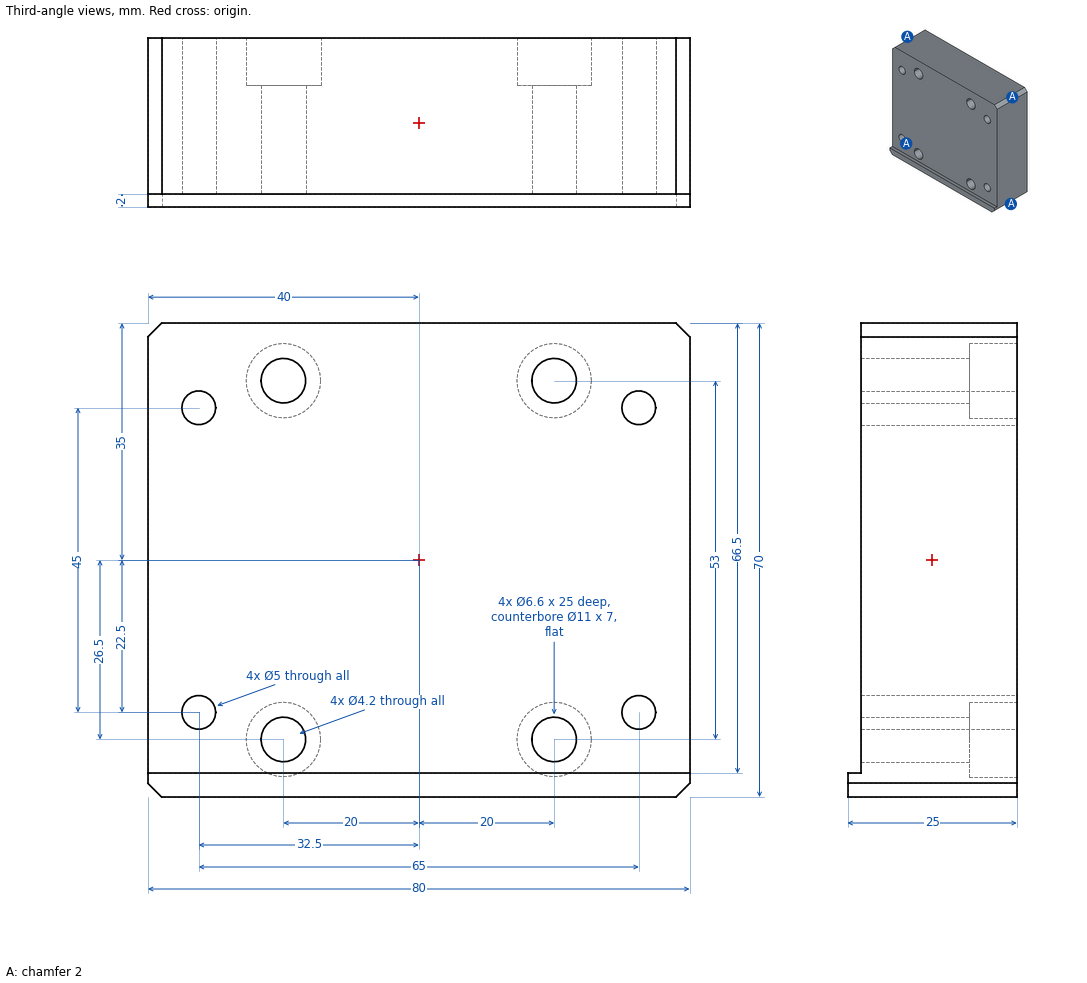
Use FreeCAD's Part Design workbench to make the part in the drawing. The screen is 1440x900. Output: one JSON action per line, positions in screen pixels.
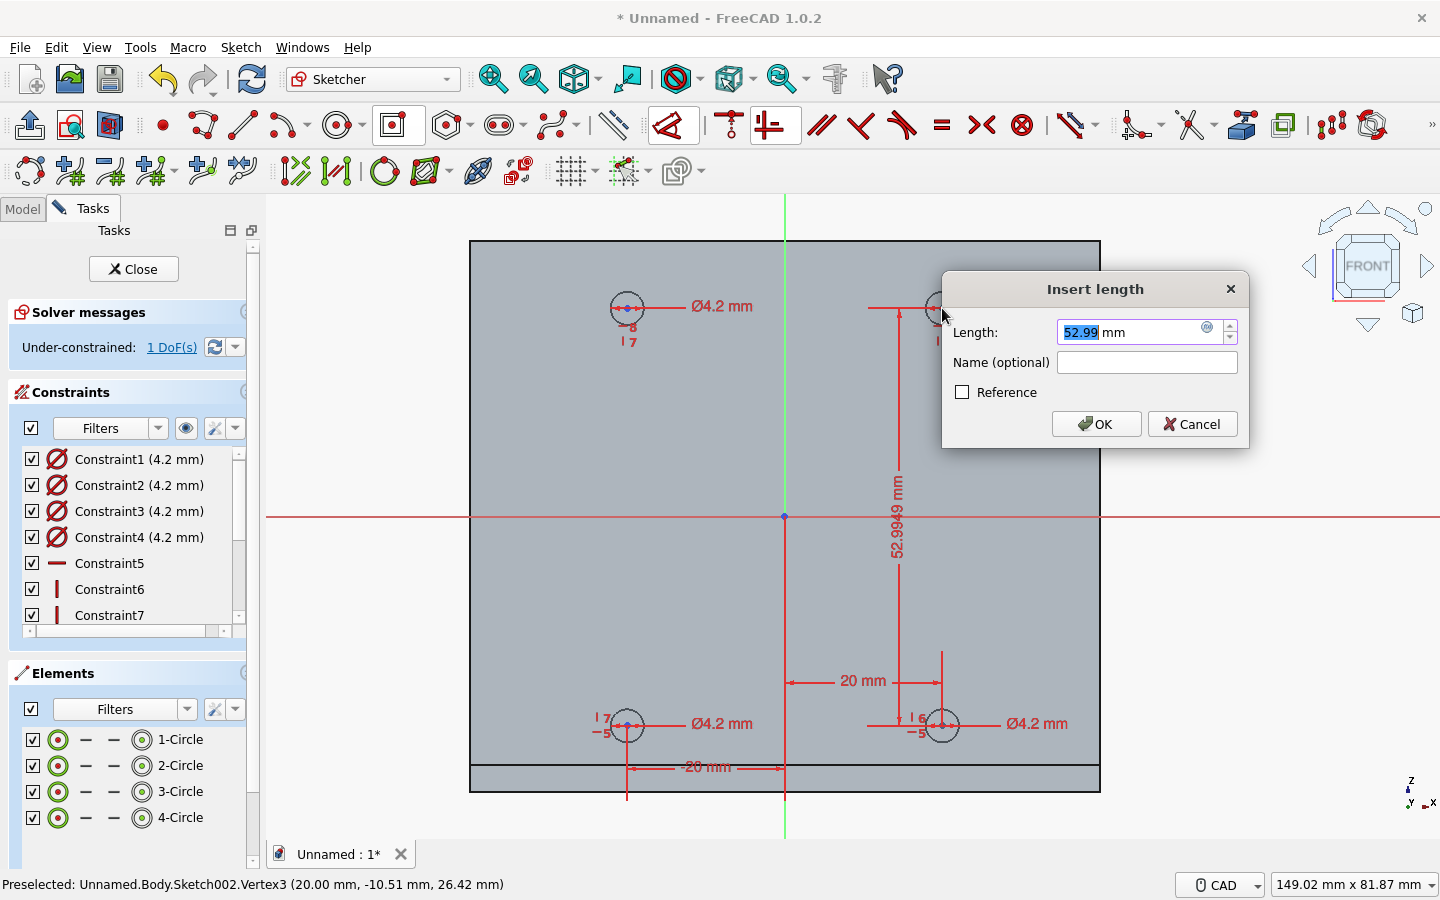
{"action": "type", "text": "53"}
{"action": "key", "text": "Return"}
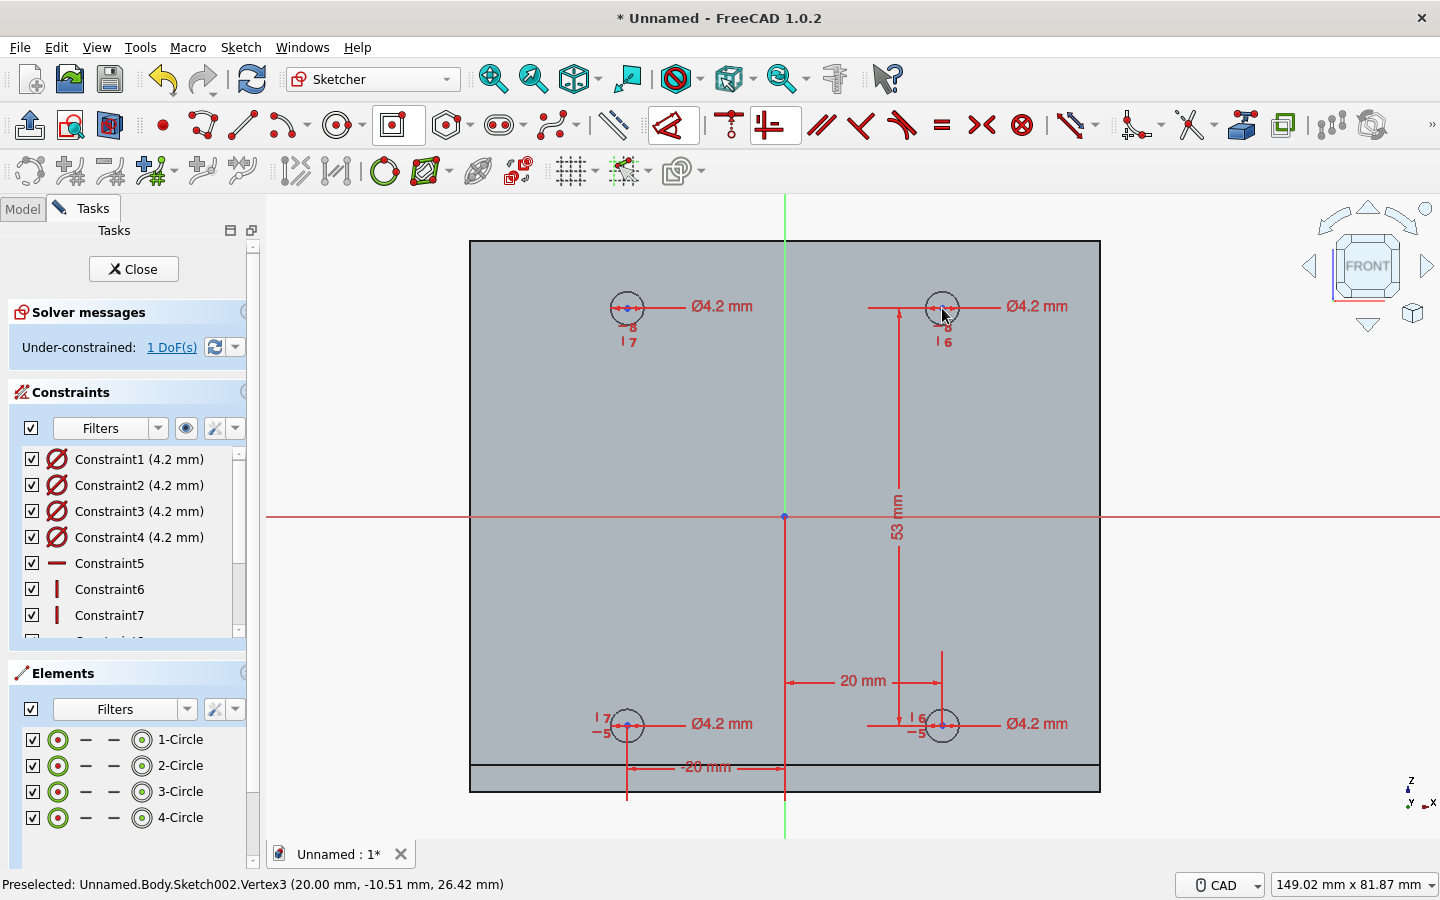
{"action": "left_click", "coordinate": [627, 726]}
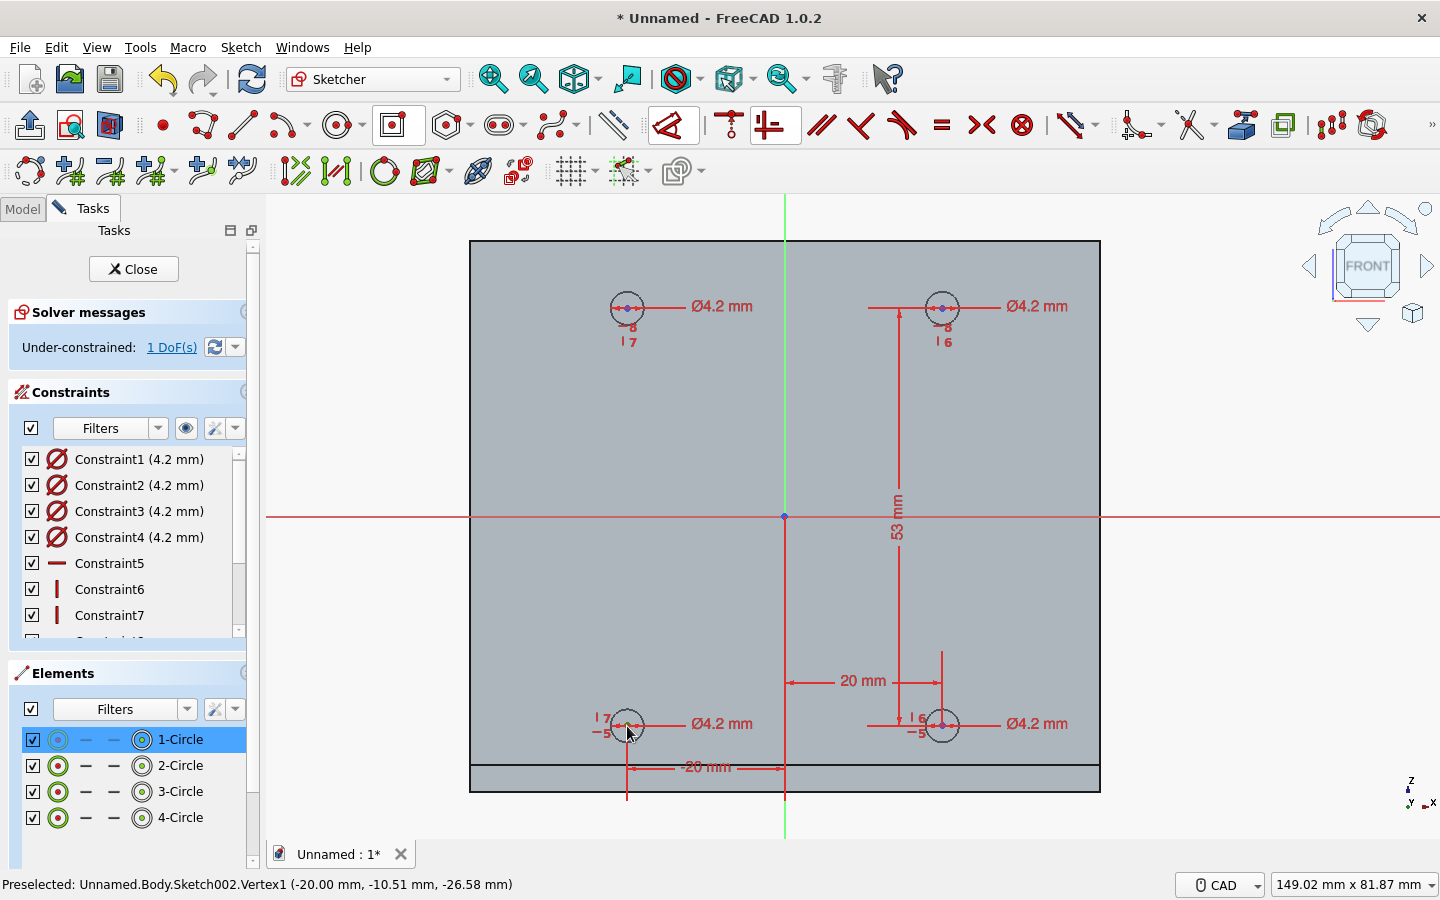
{"action": "left_click", "coordinate": [694, 126]}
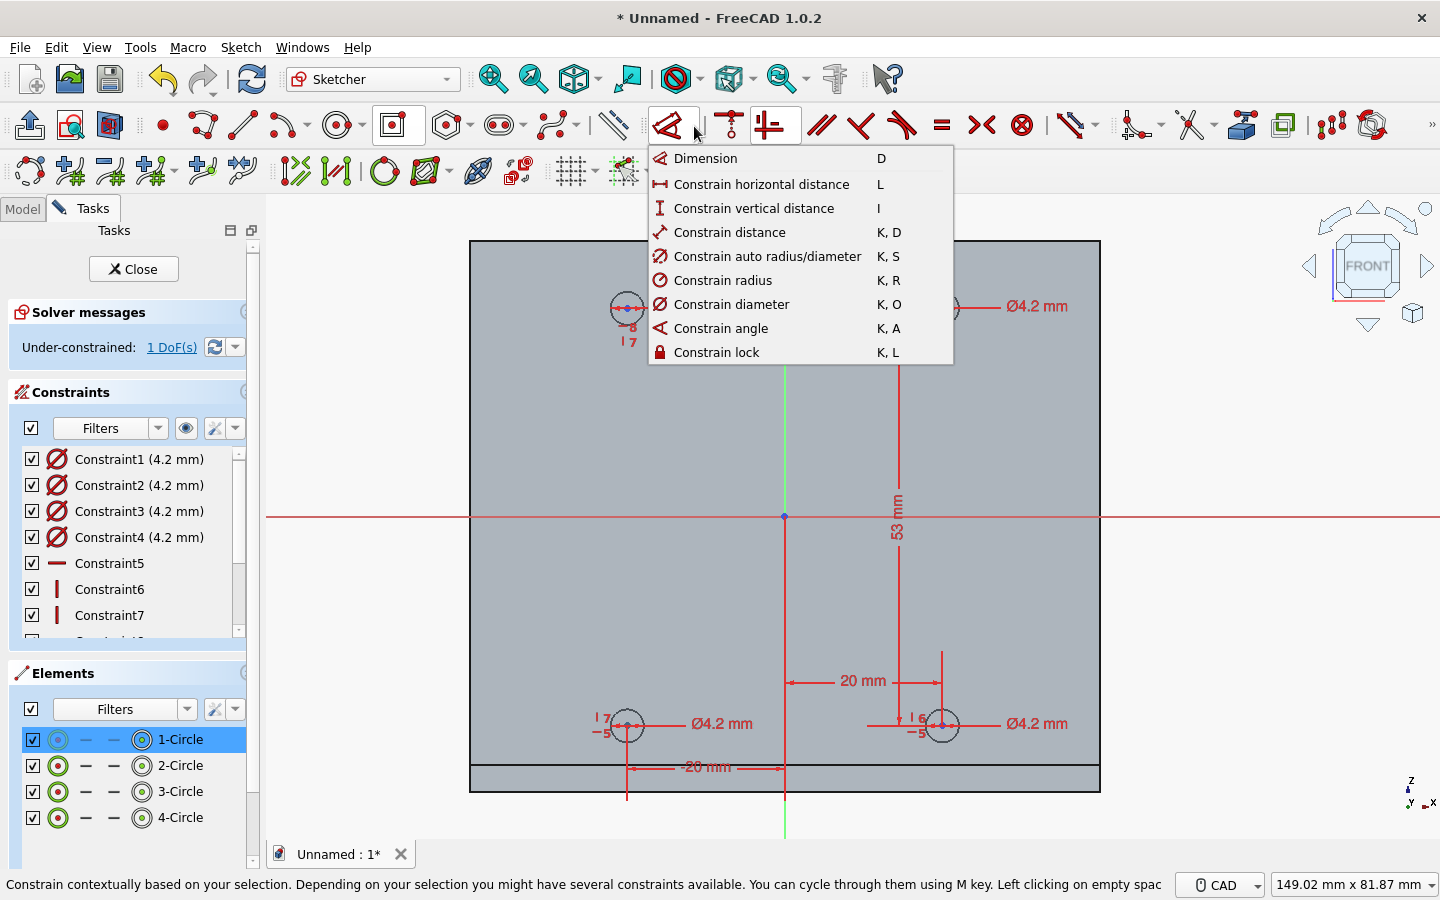
{"action": "left_click", "coordinate": [801, 208]}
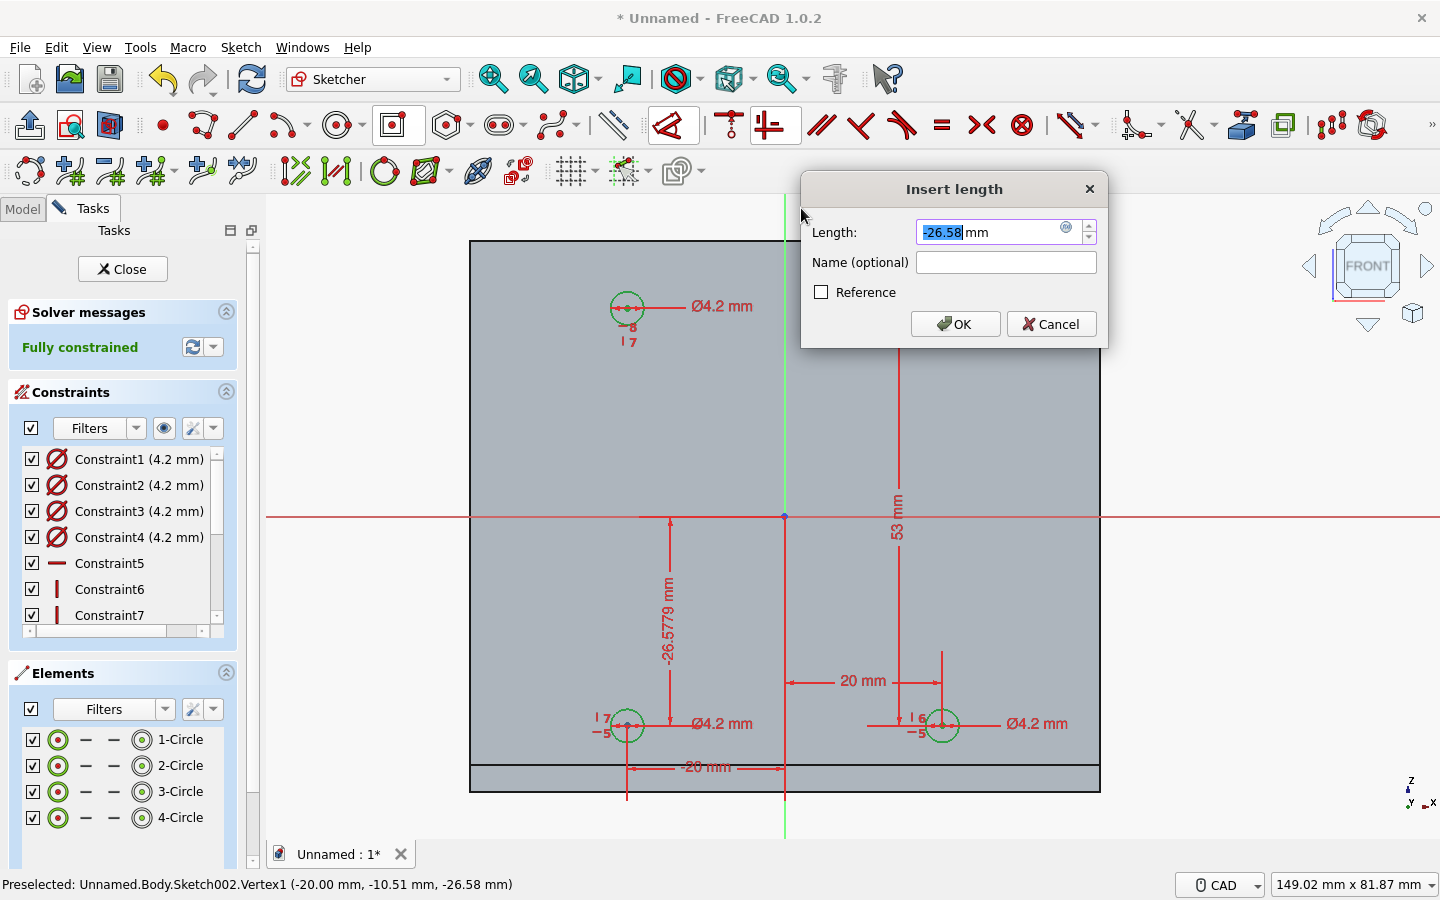
{"action": "type", "text": "-26.5"}
{"action": "key", "text": "Return"}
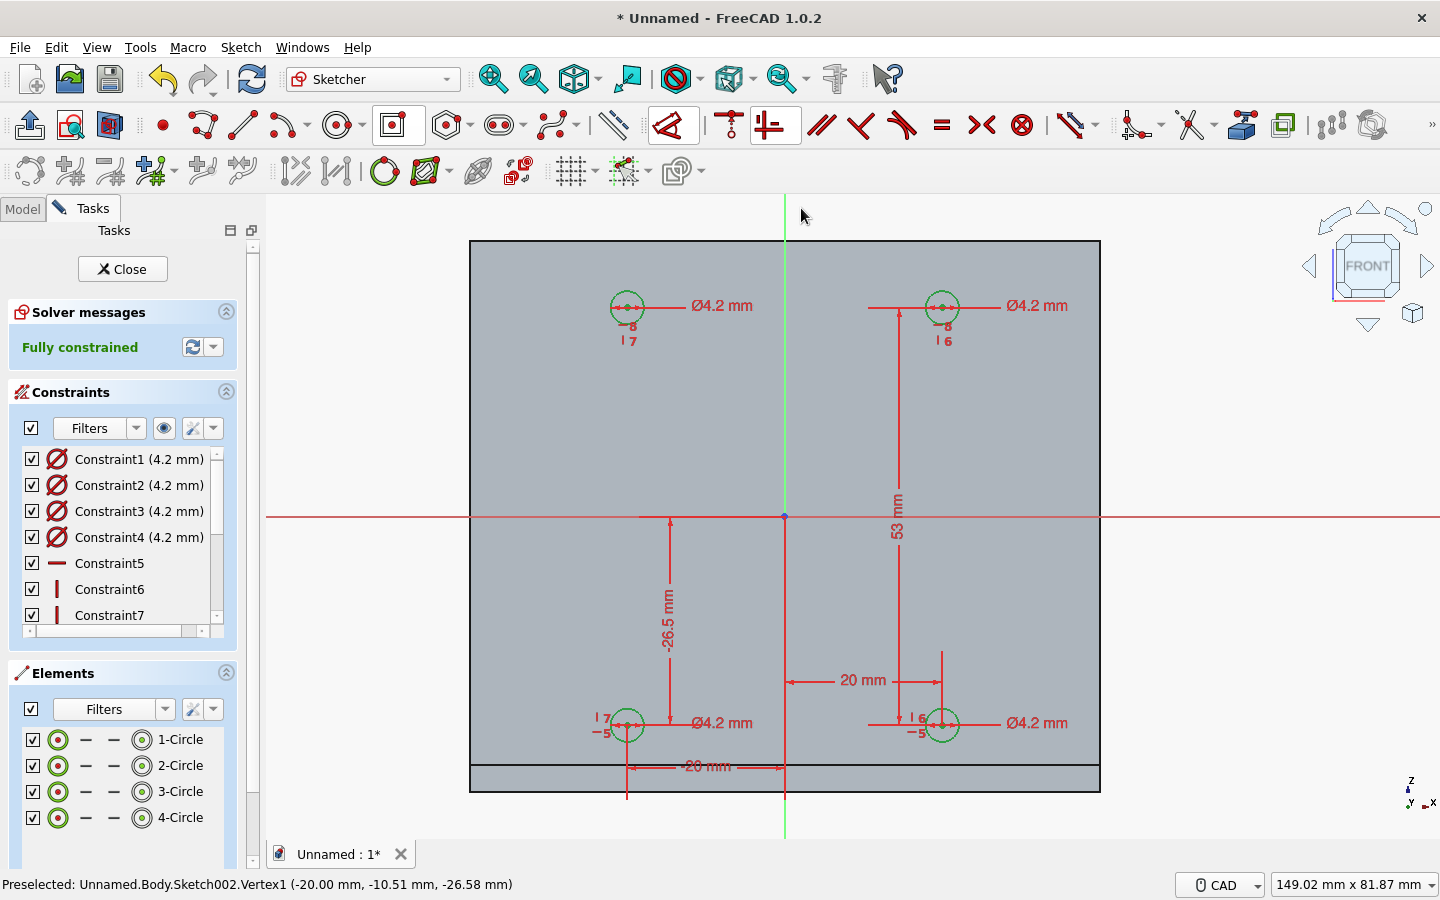
{"action": "left_click", "coordinate": [123, 269]}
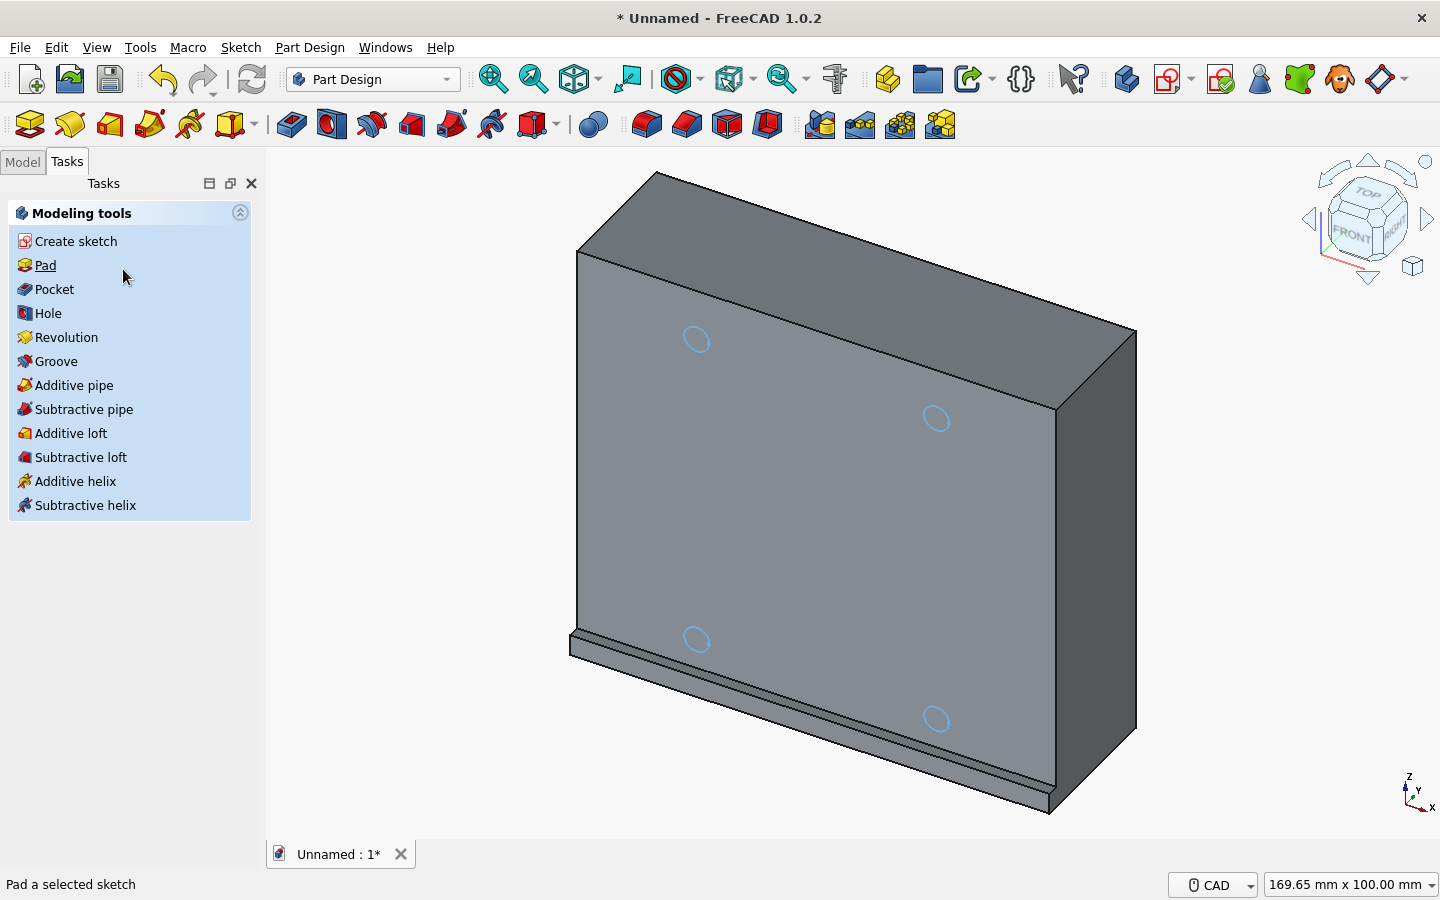
{"action": "left_click", "coordinate": [332, 124]}